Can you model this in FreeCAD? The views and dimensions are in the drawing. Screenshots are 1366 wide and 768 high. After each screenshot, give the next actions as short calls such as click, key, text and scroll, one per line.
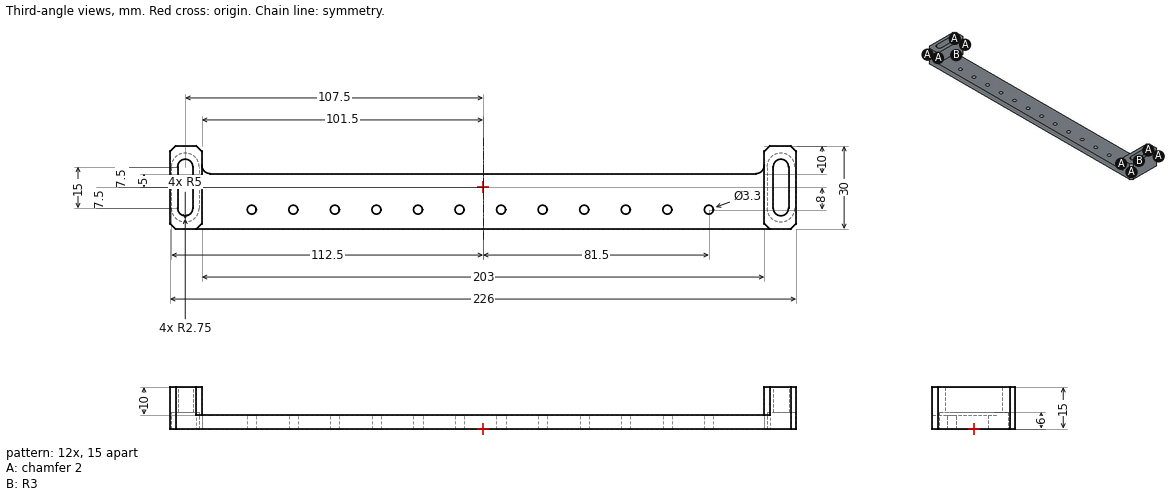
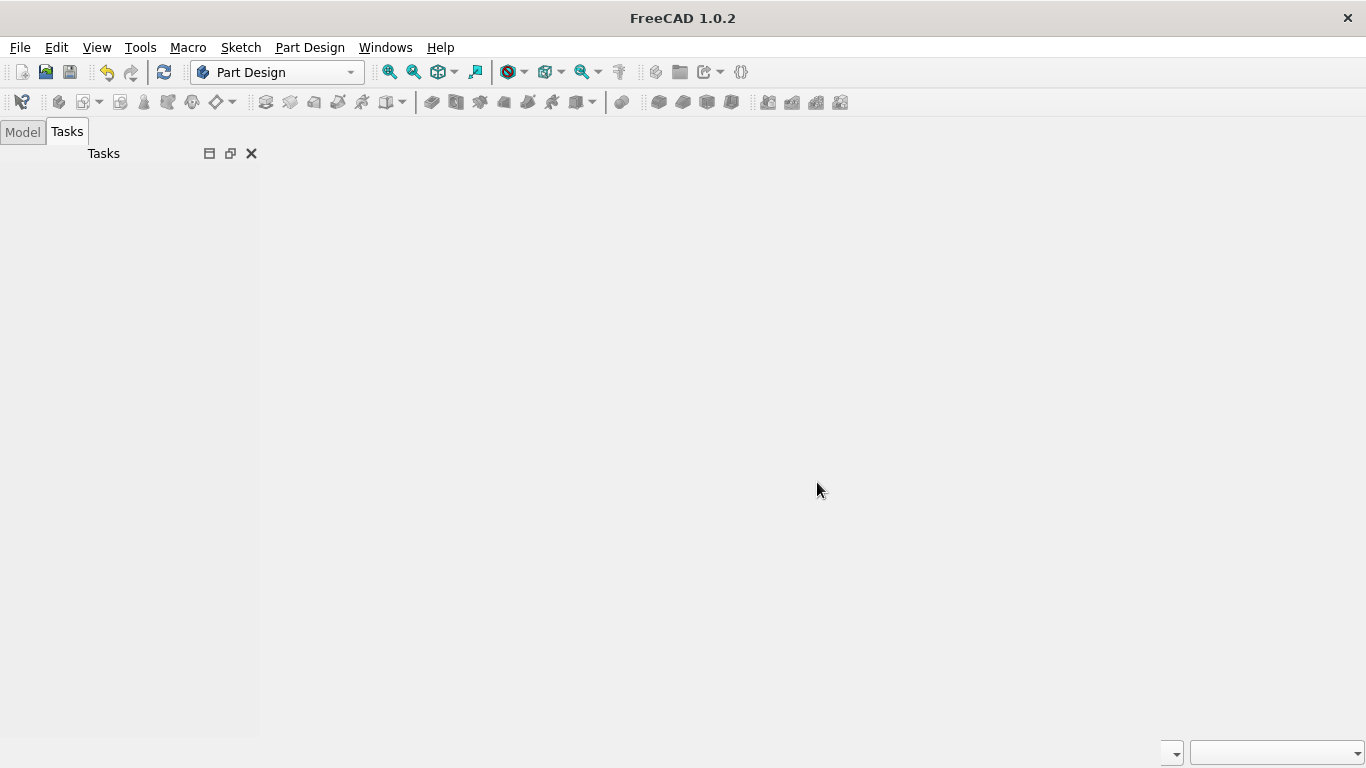
click(22, 72)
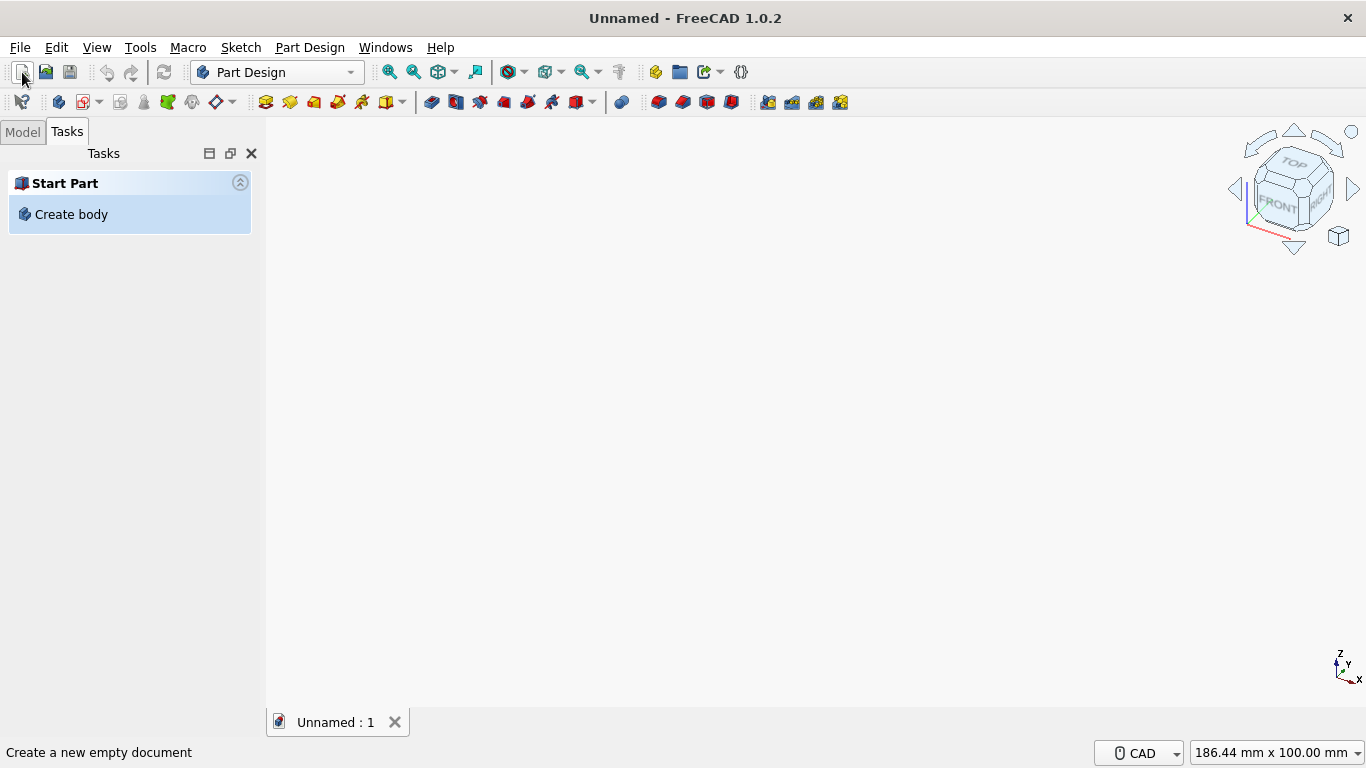
click(84, 102)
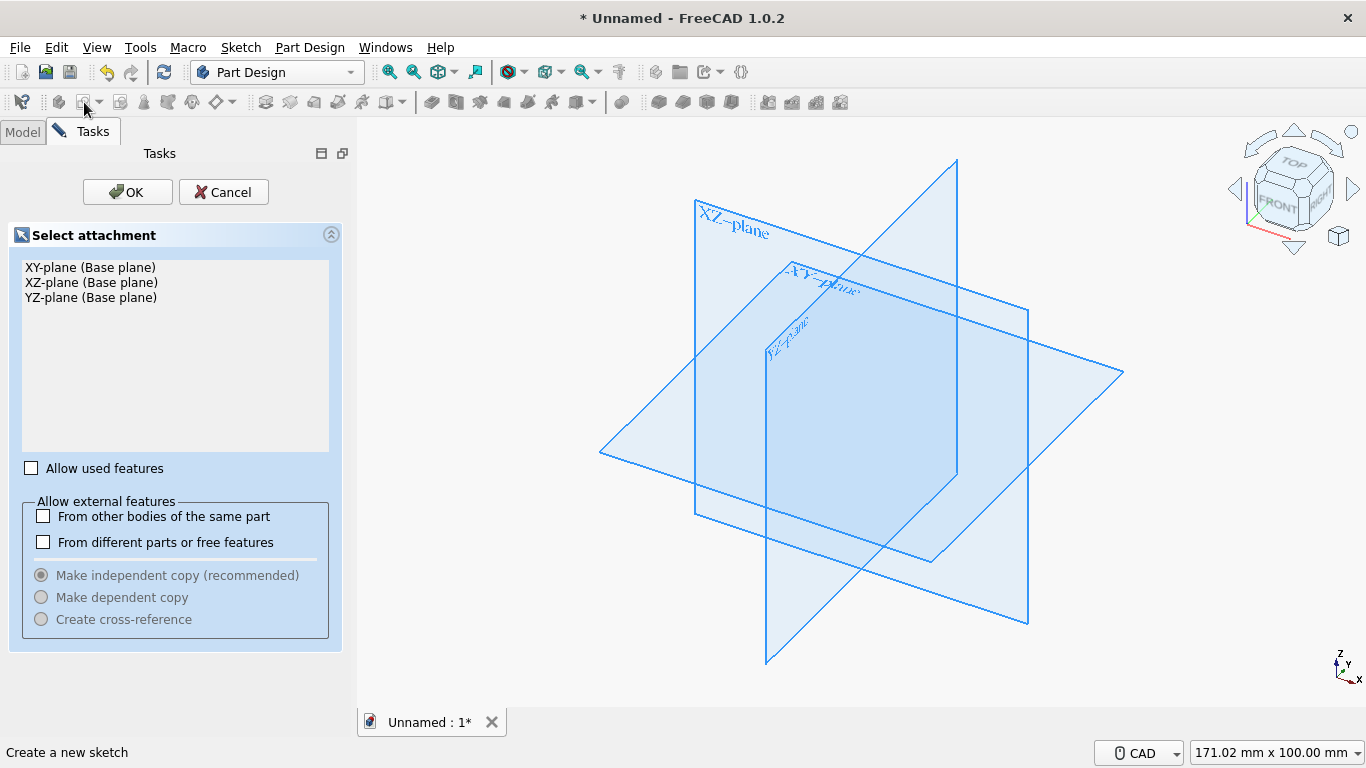
click(82, 268)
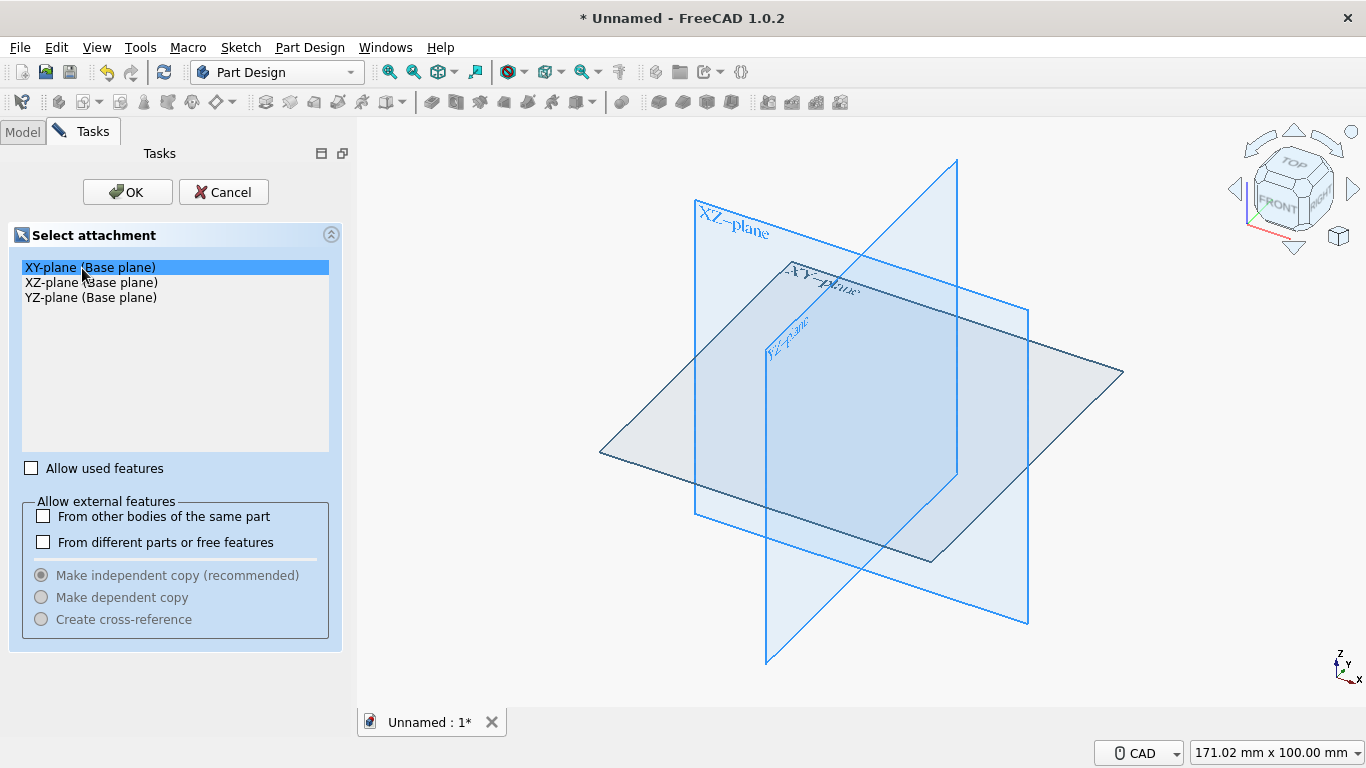
click(128, 192)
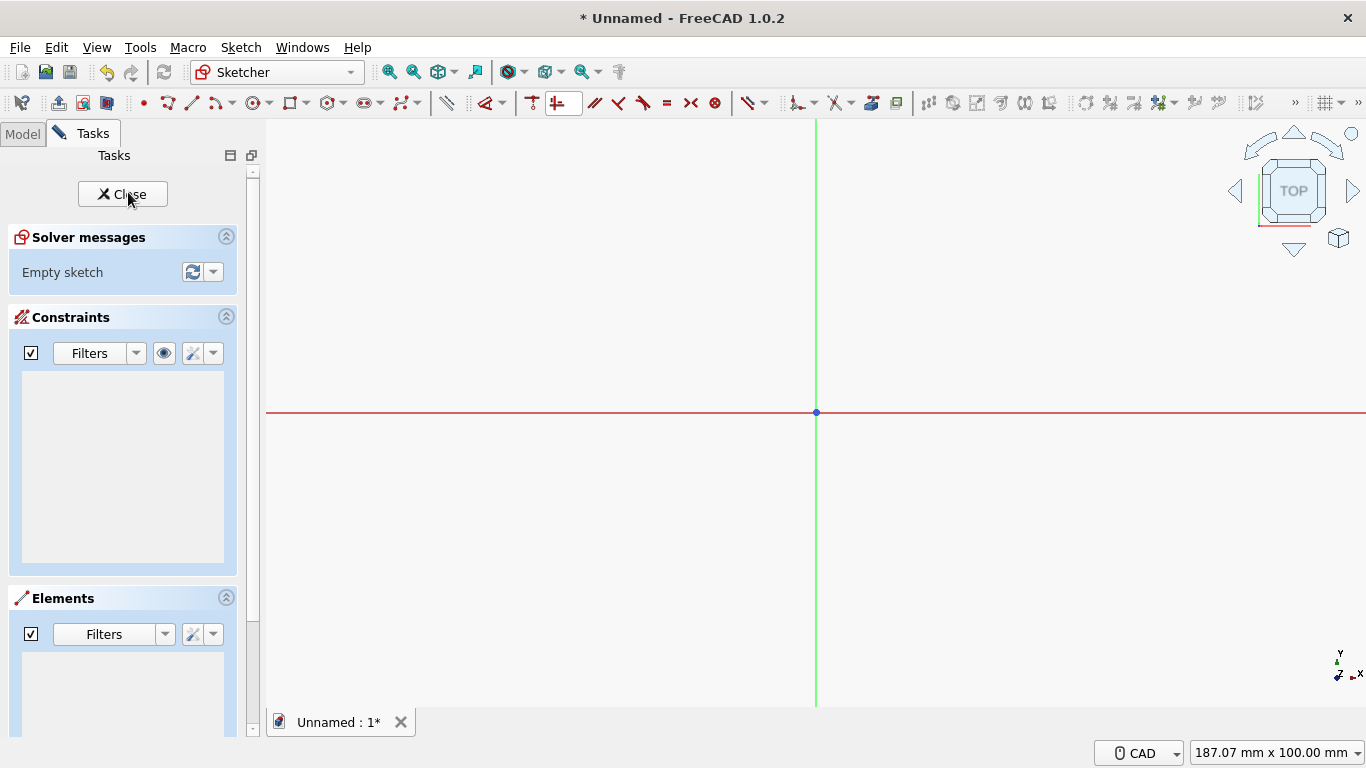
scroll(692, 413, down, 4)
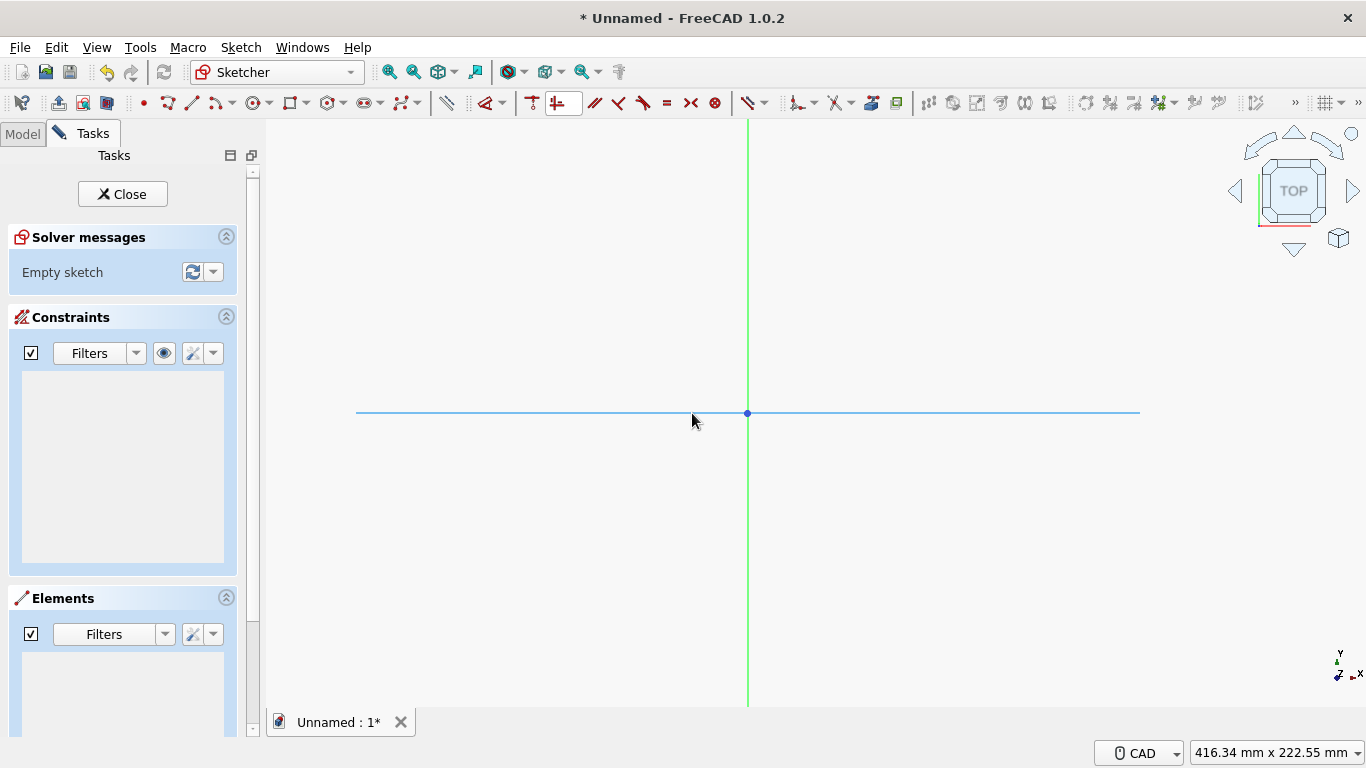
key(g)
key(v)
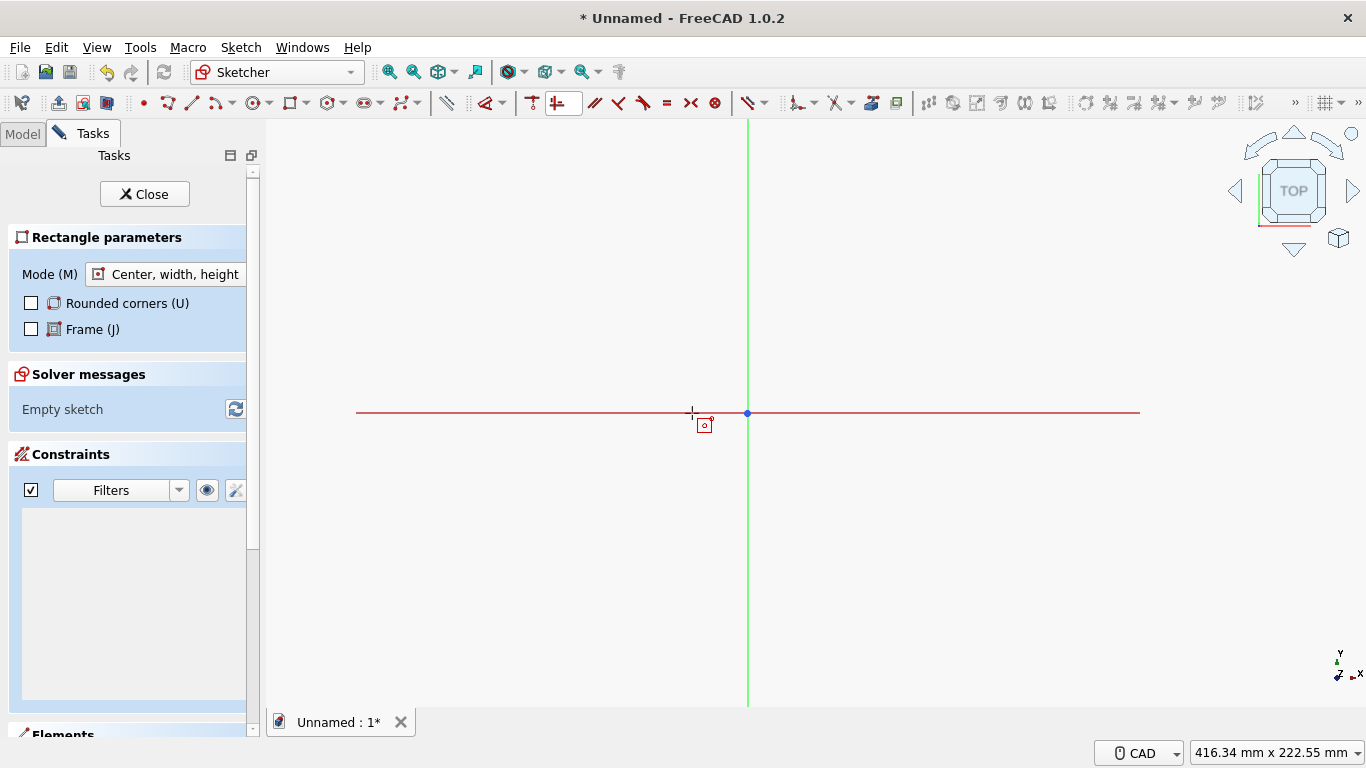
click(748, 413)
move(1046, 374)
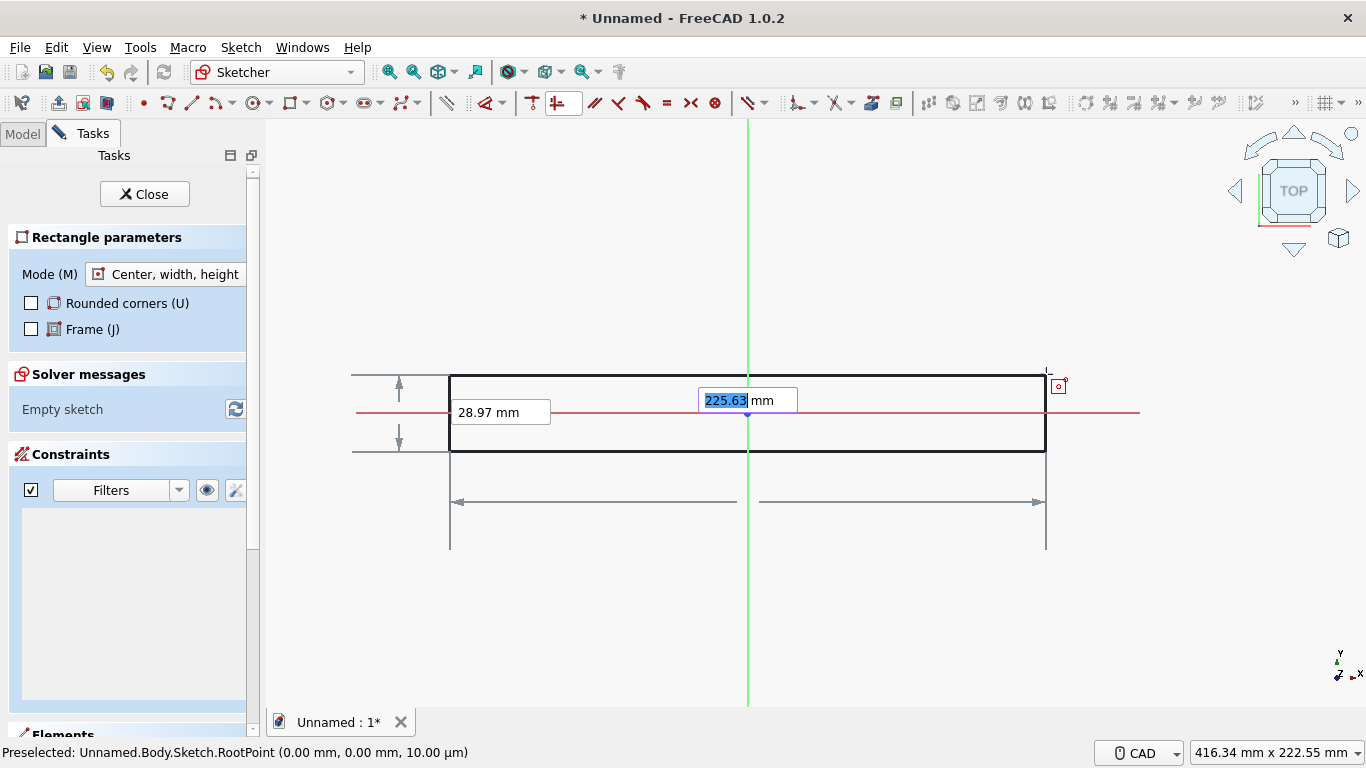
text(226)
key(Tab)
text(30)
key(Return)
key(Escape)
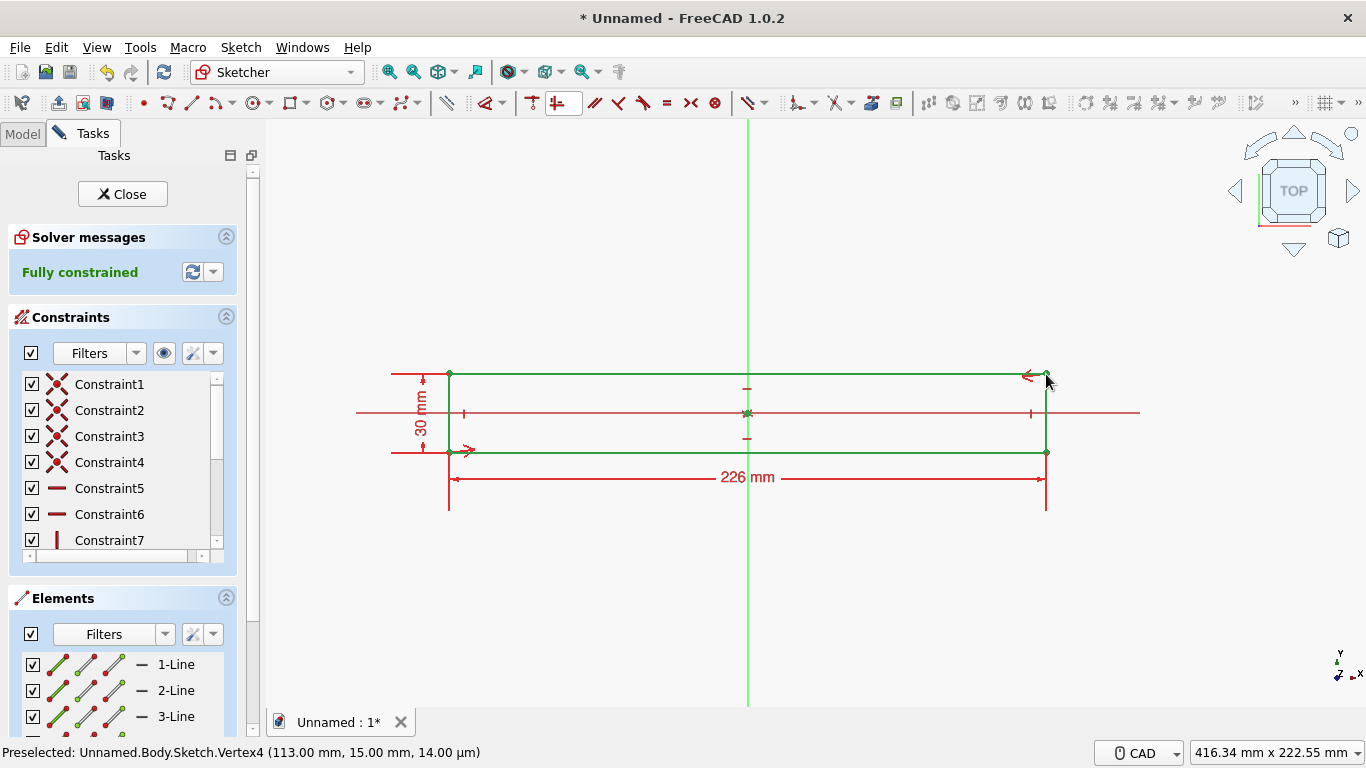
click(123, 194)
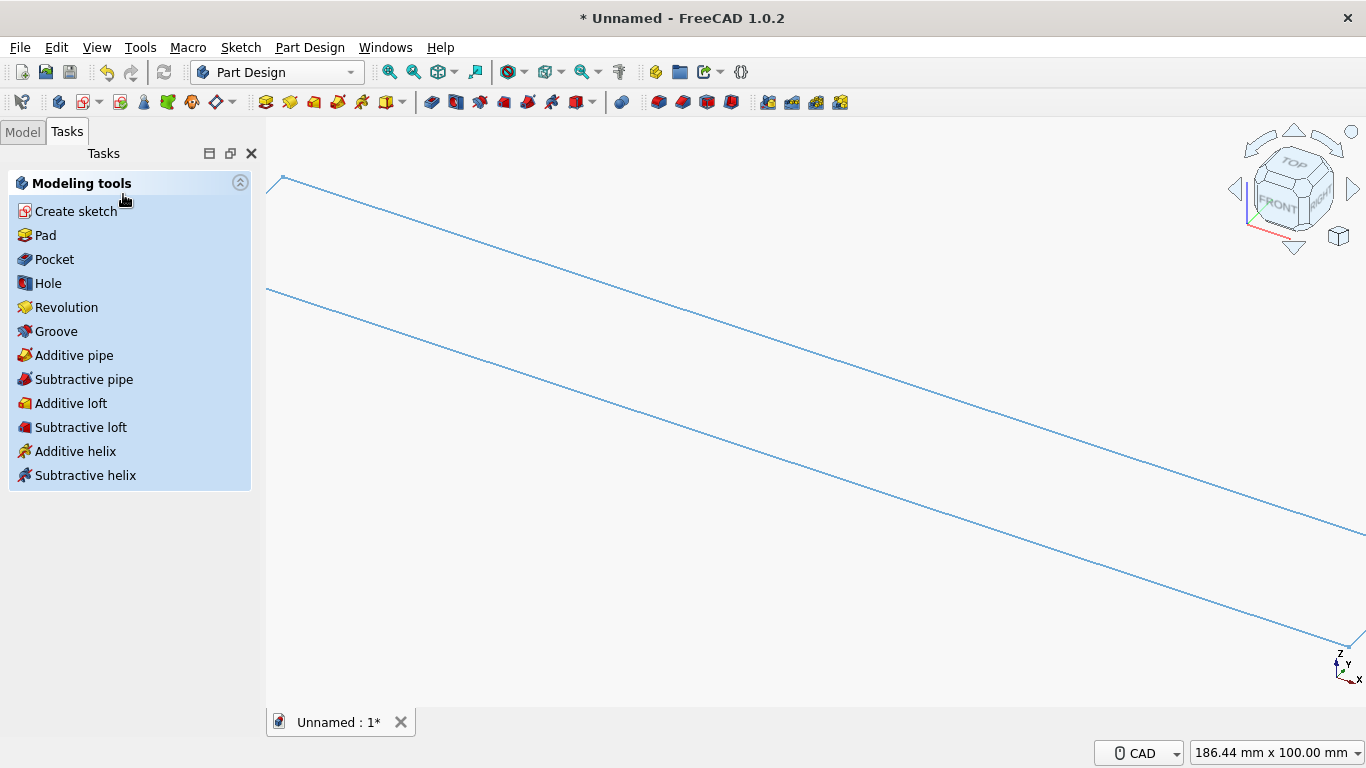
click(266, 102)